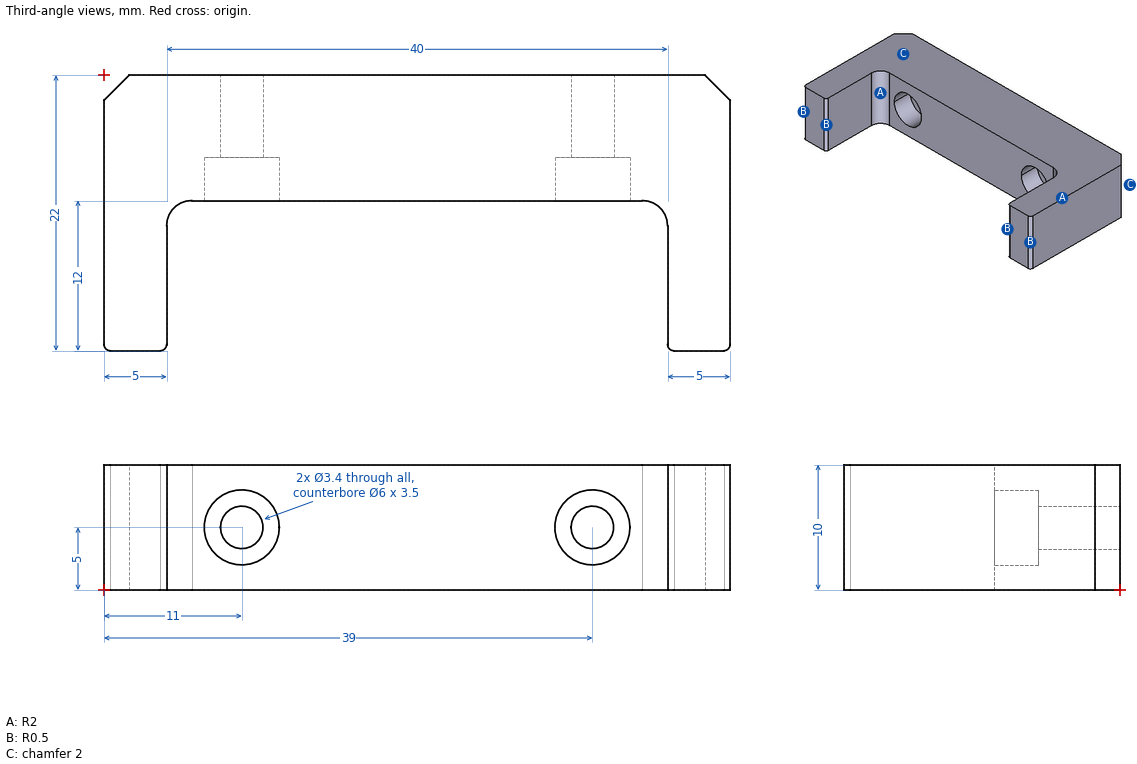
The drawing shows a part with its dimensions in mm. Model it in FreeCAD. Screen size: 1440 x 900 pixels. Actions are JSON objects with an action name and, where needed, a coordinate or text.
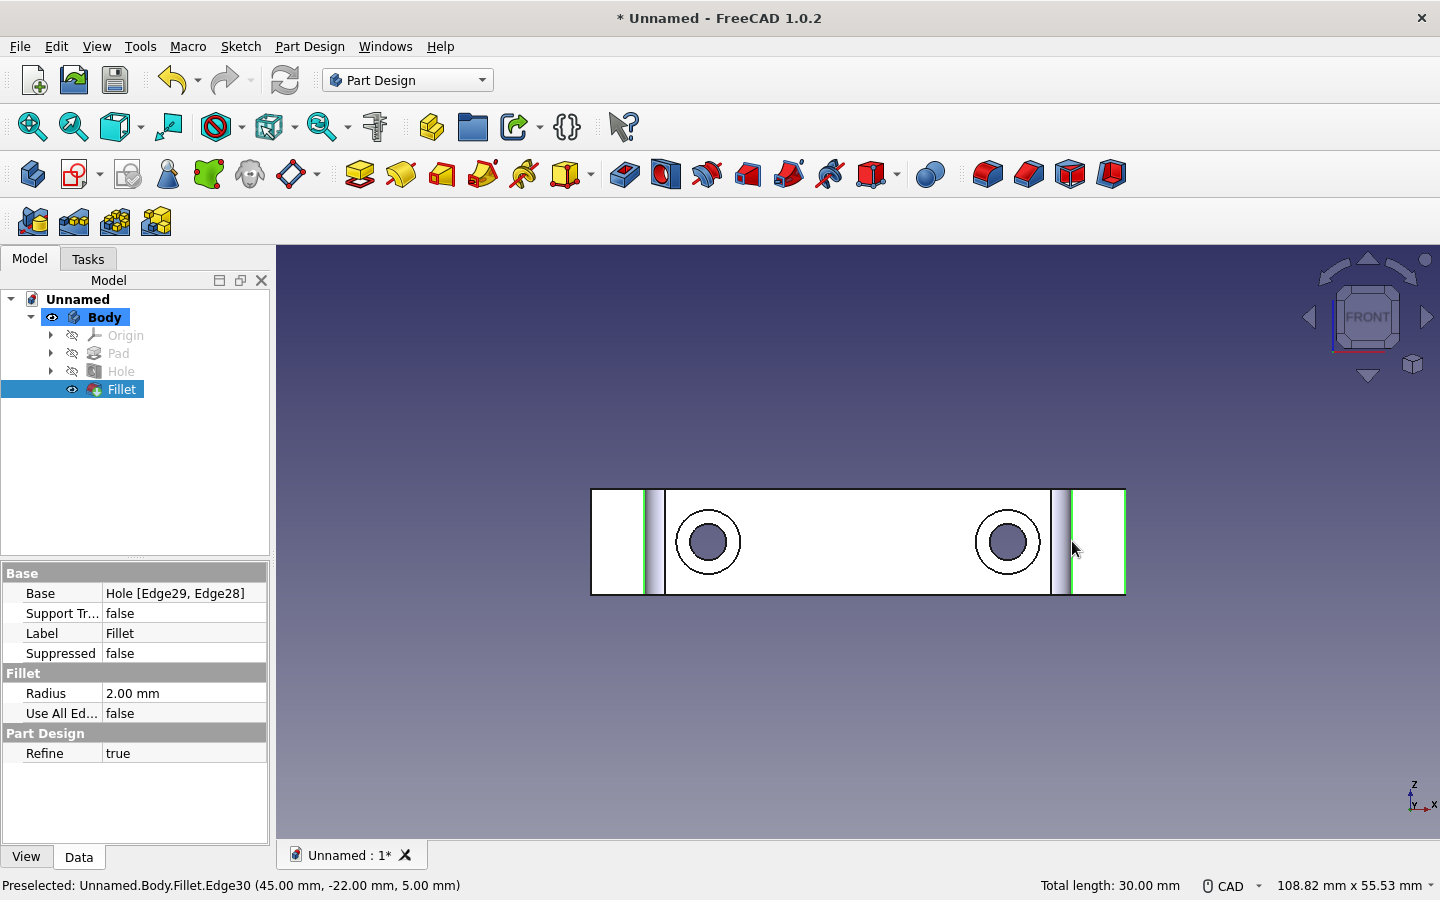
{"action": "left_click", "coordinate": [591, 541], "text": "ctrl"}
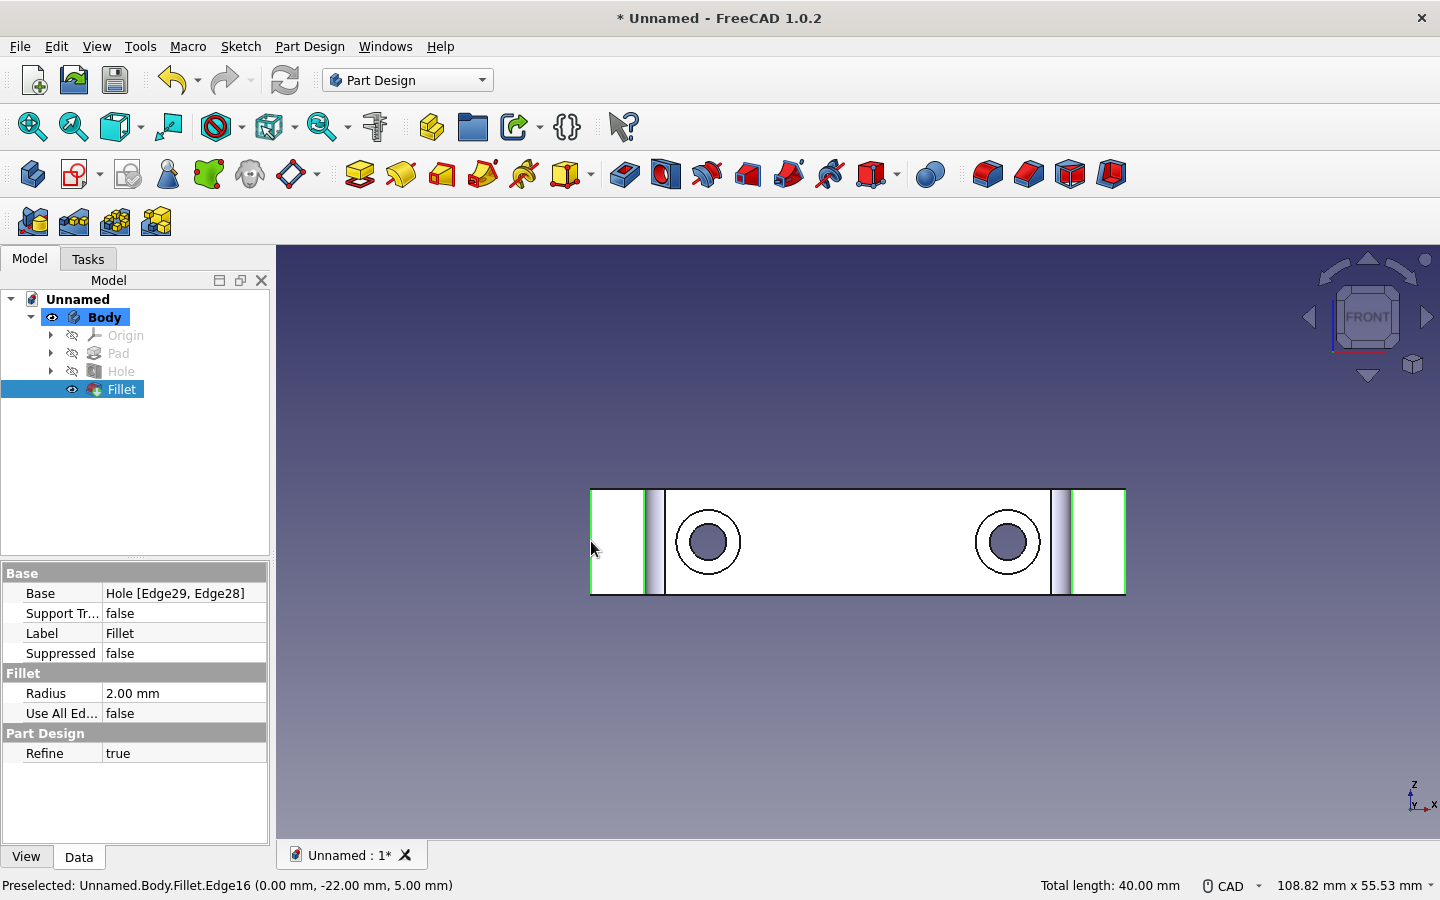
{"action": "left_click", "coordinate": [988, 174]}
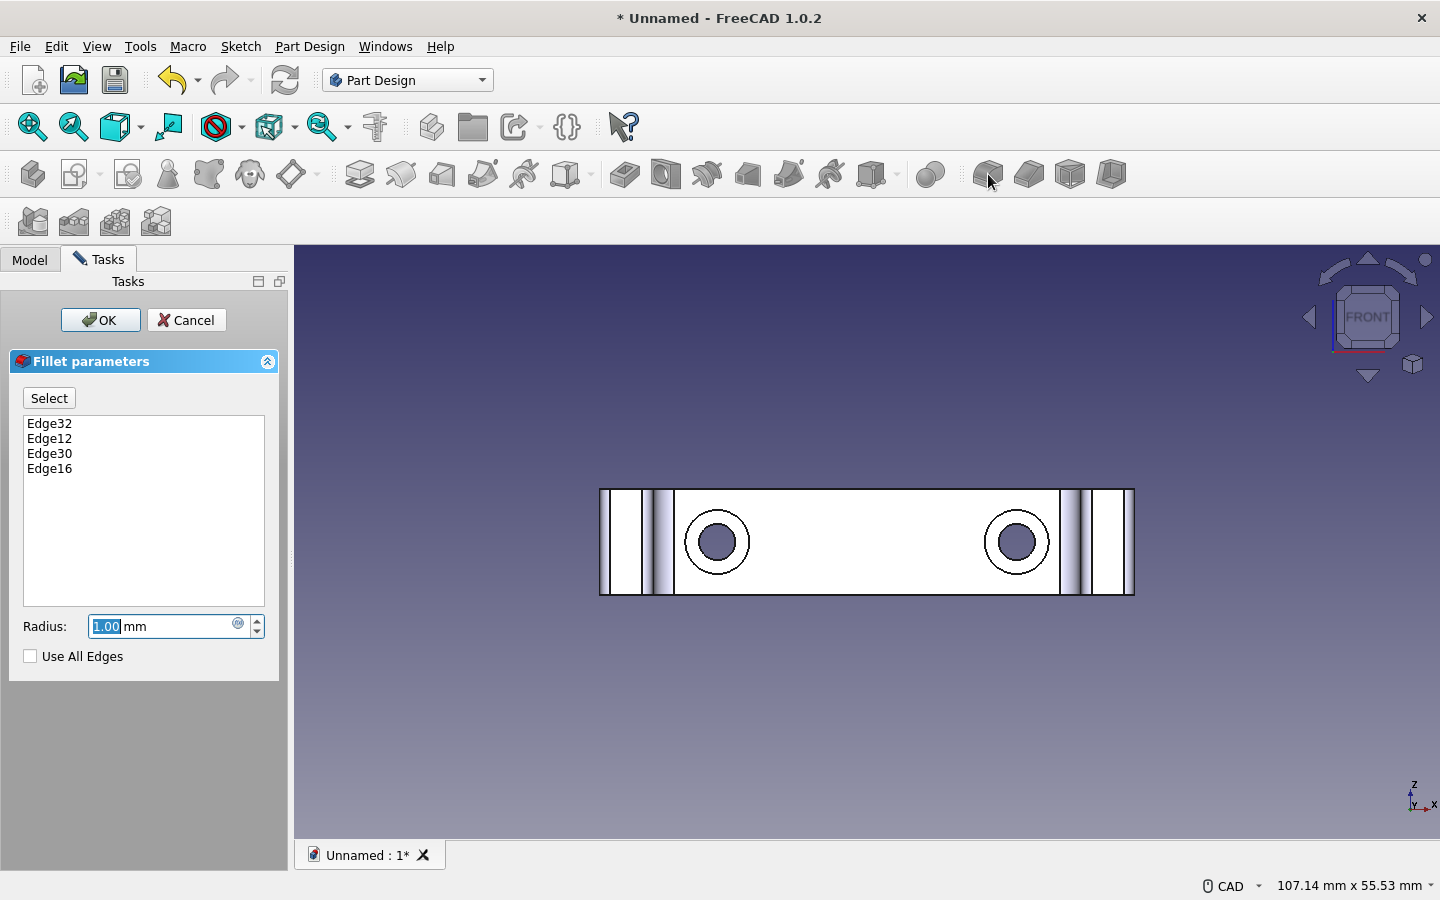
{"action": "type", "text": "0.5"}
{"action": "key", "text": "Tab"}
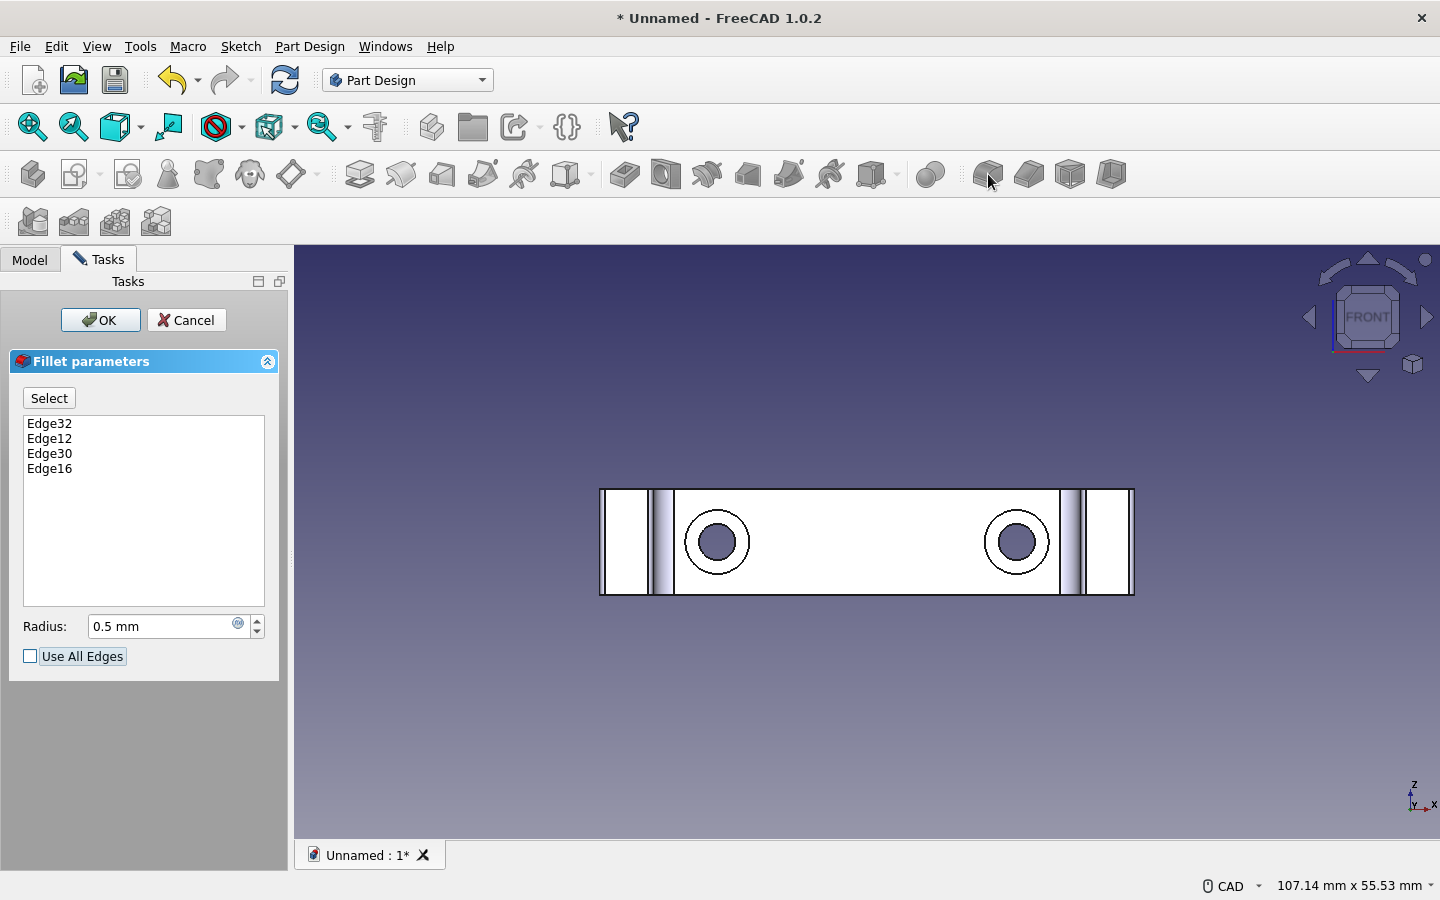
{"action": "left_click", "coordinate": [101, 320]}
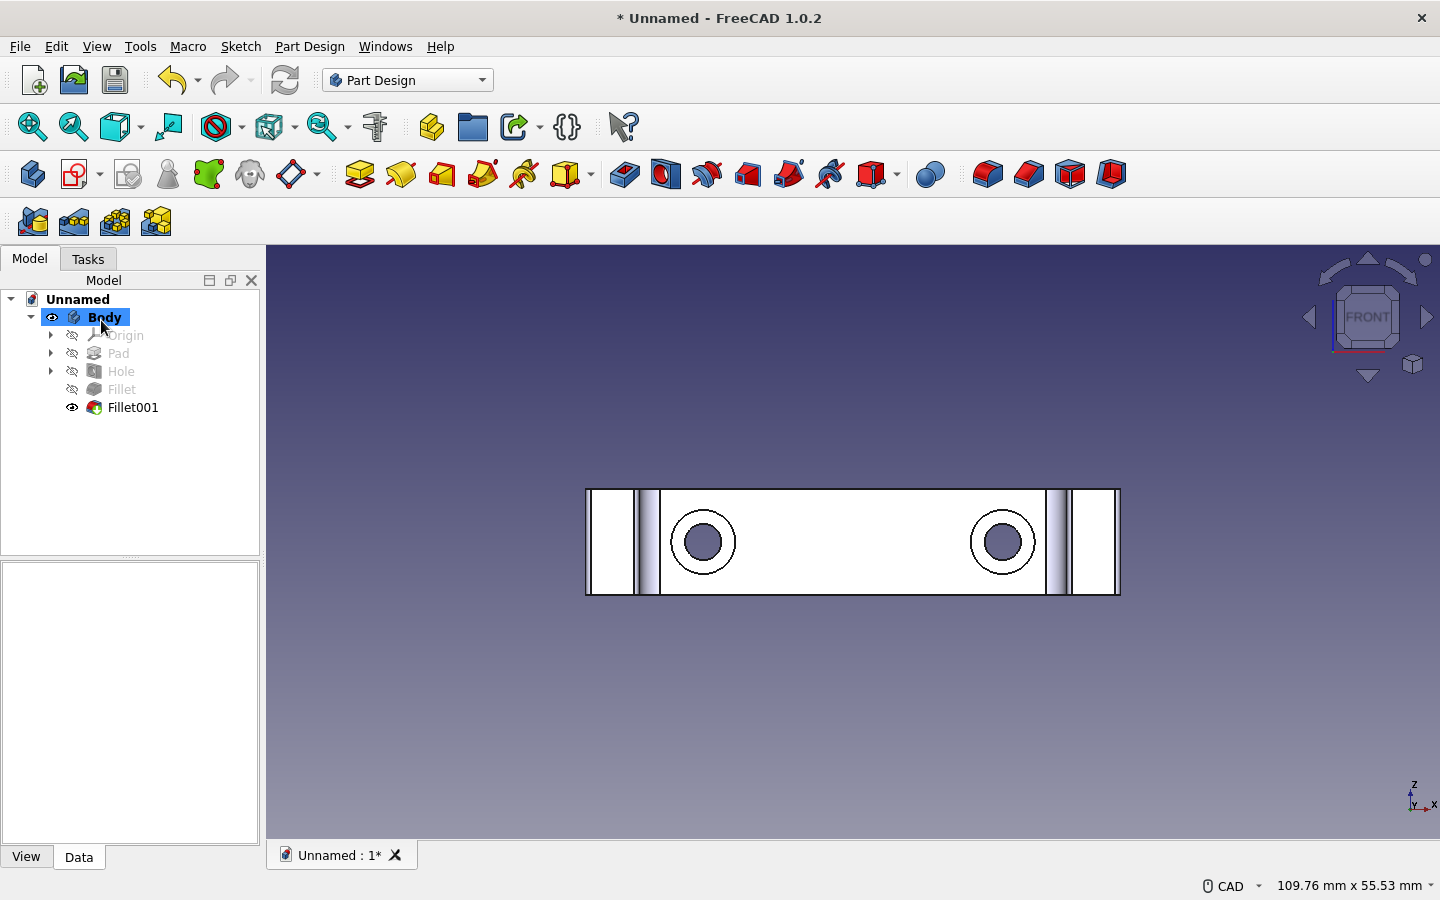
{"action": "key", "text": "0"}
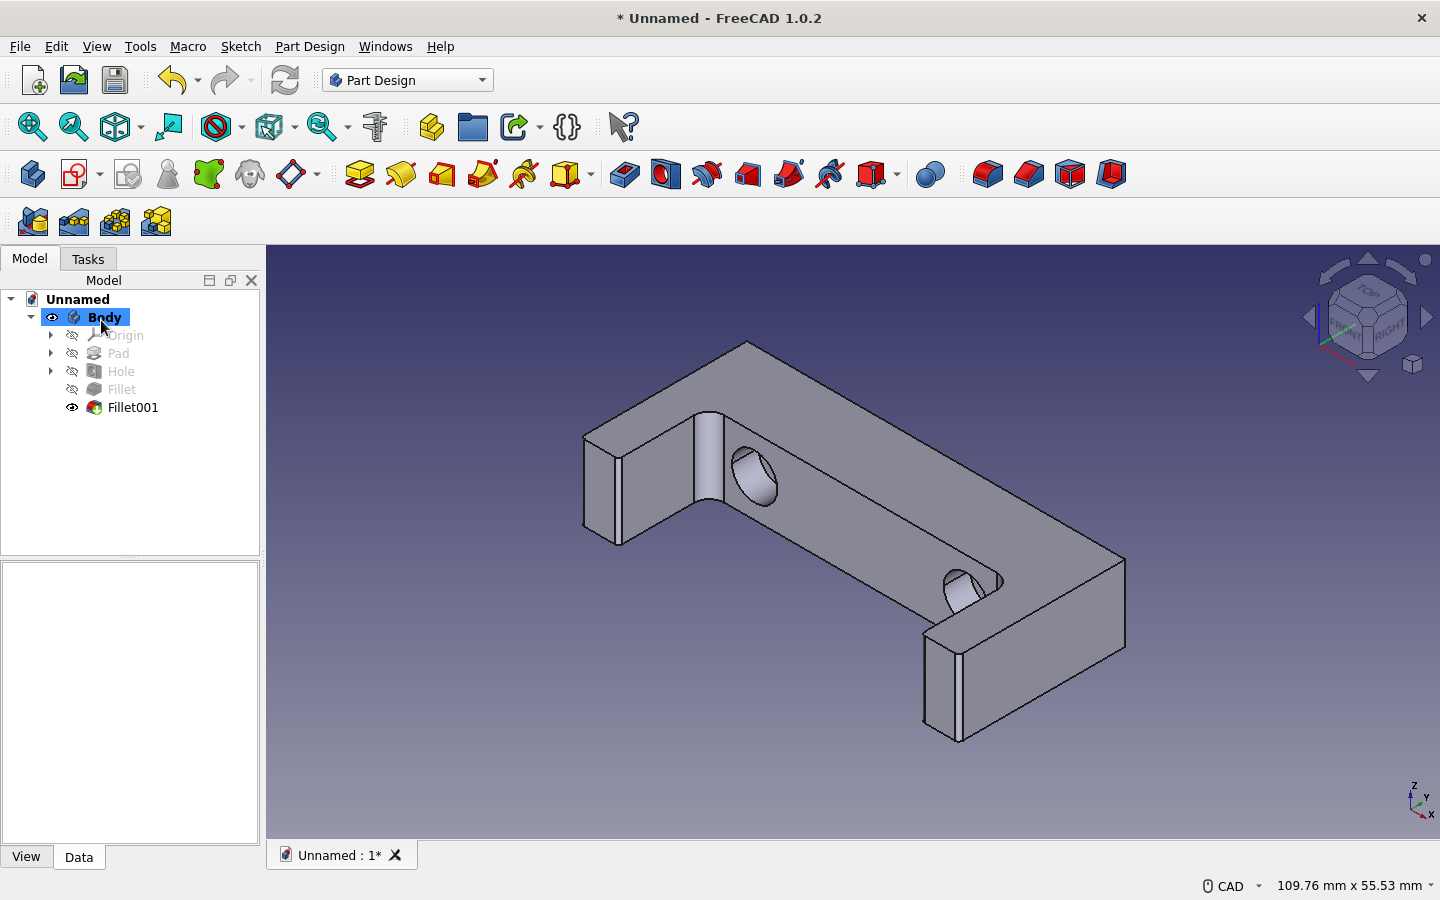
{"action": "key", "text": "2"}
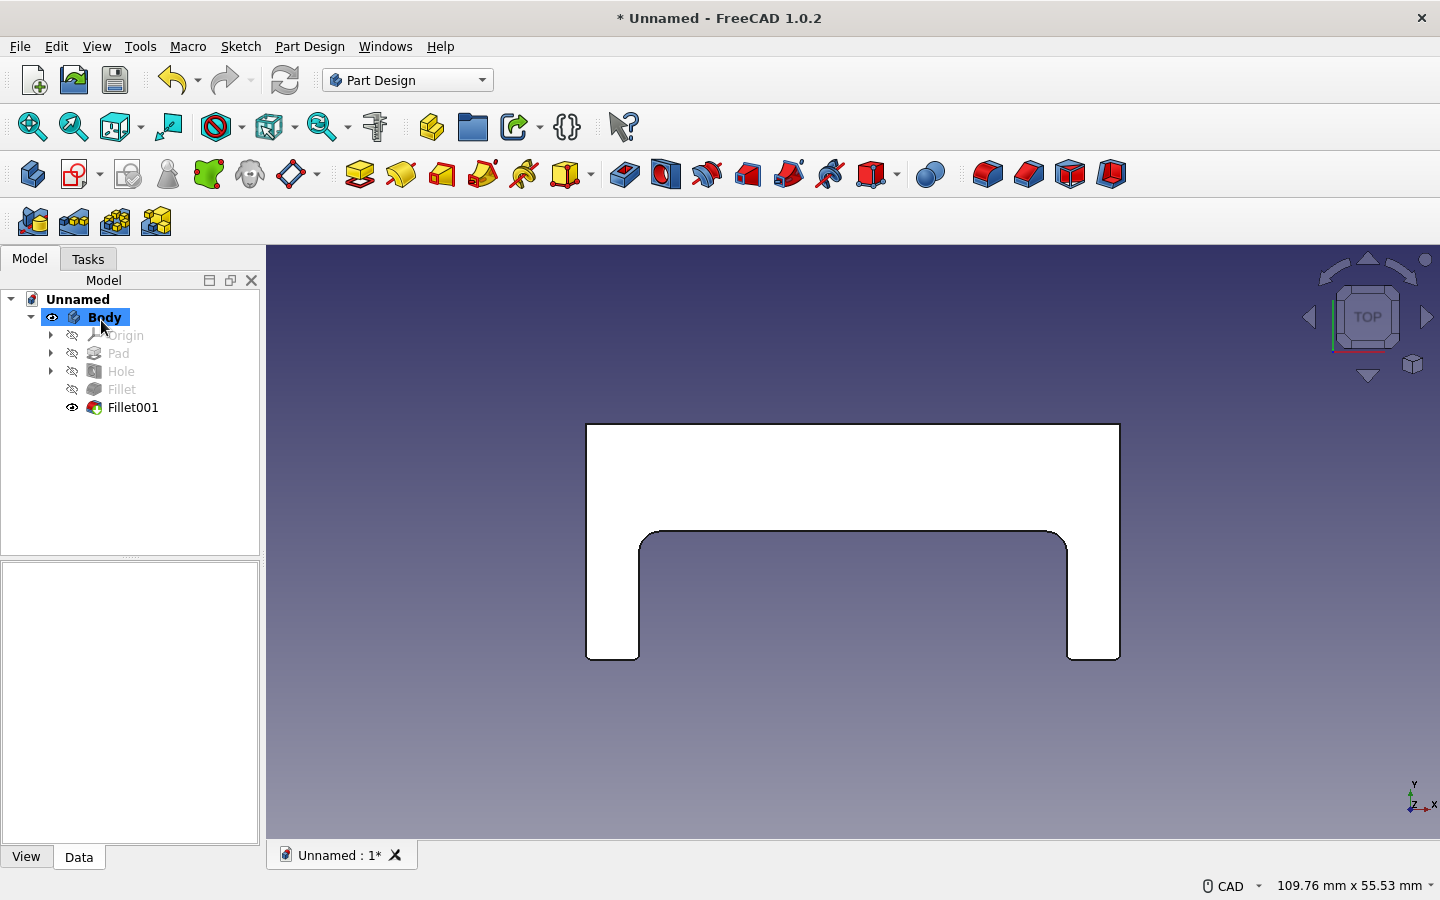
{"action": "key", "text": "1"}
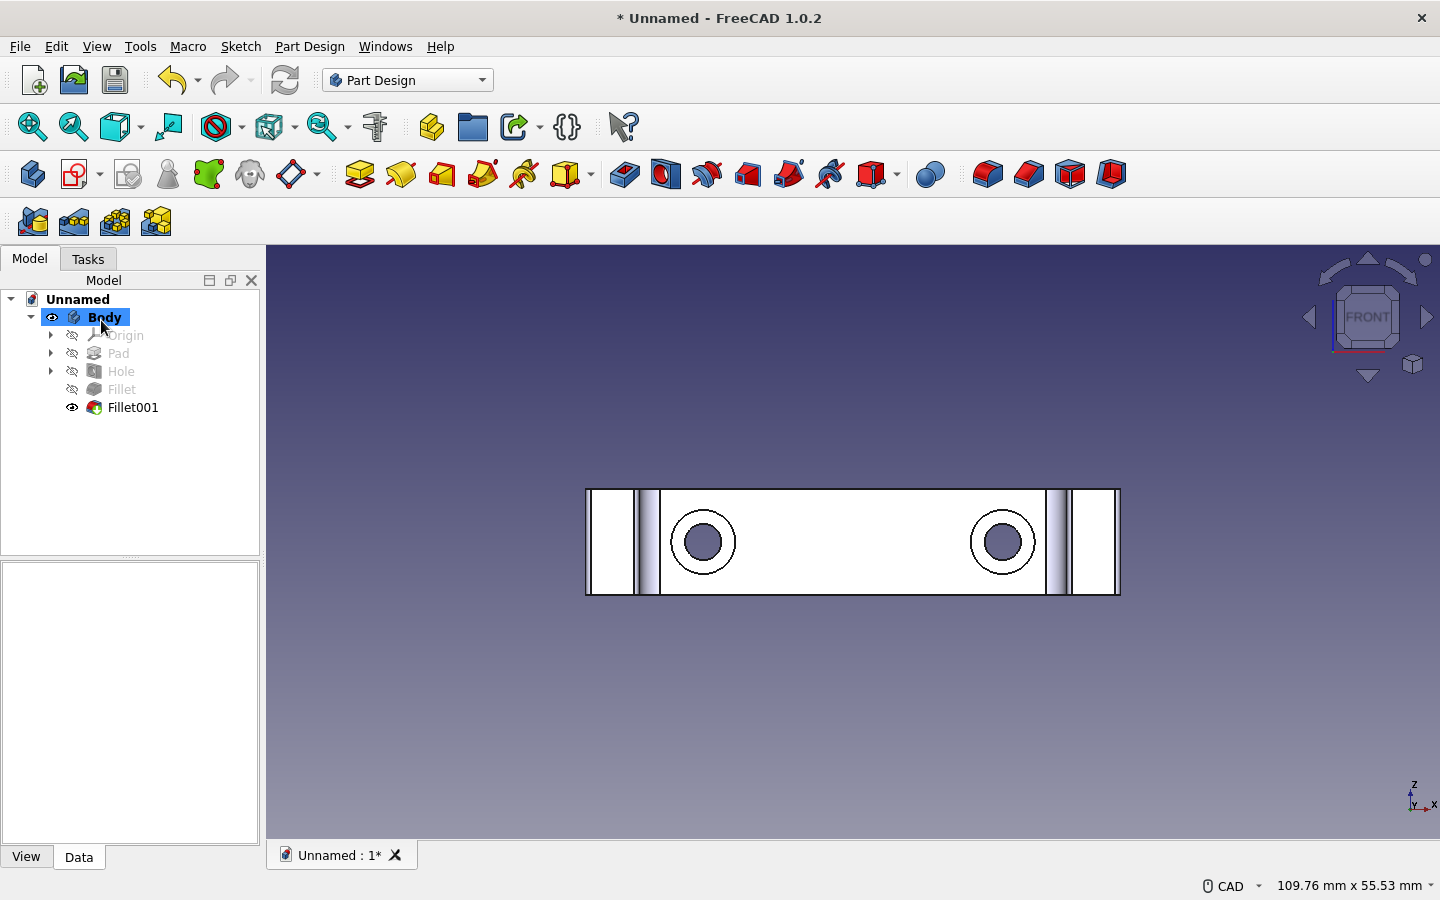
{"action": "key", "text": "3"}